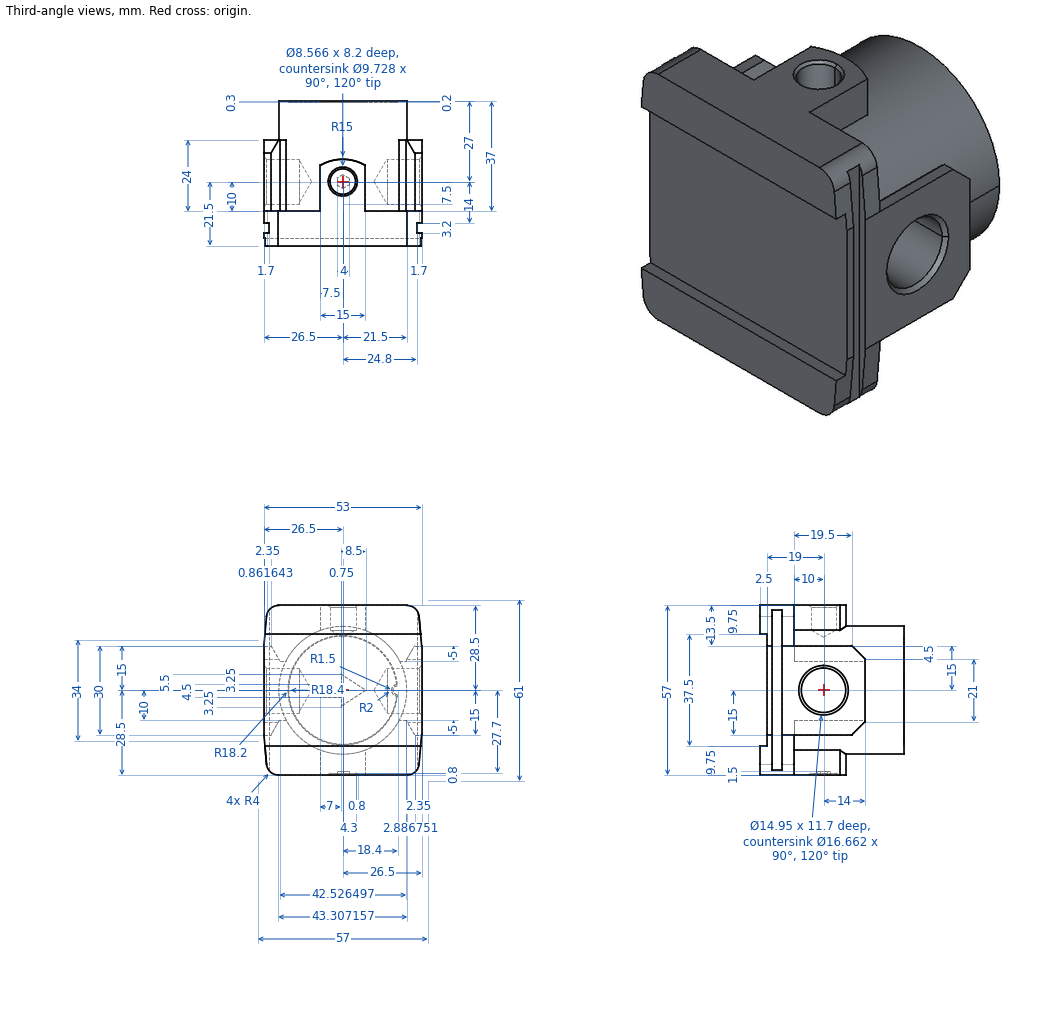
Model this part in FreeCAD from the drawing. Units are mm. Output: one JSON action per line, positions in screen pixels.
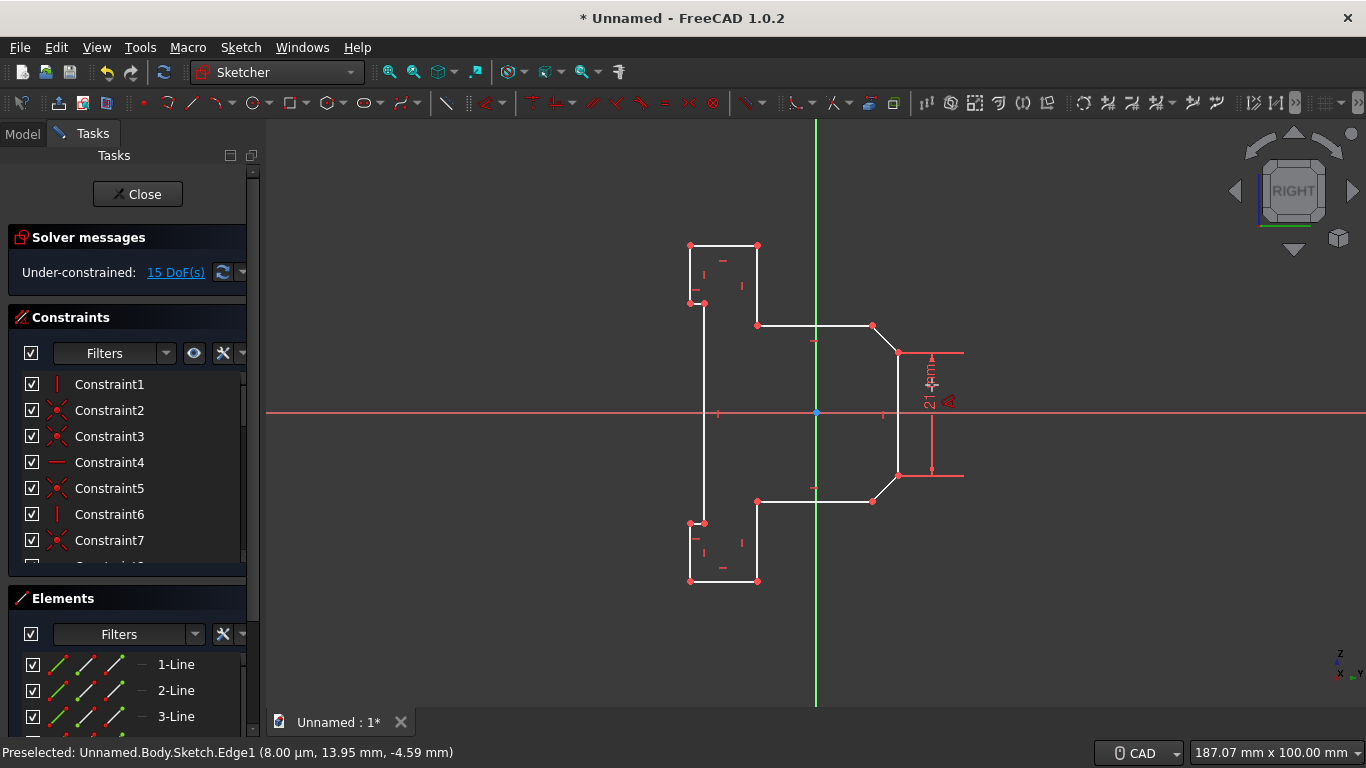
{"action": "scroll", "coordinate": [697, 304], "scroll_direction": "up", "scroll_amount": 5}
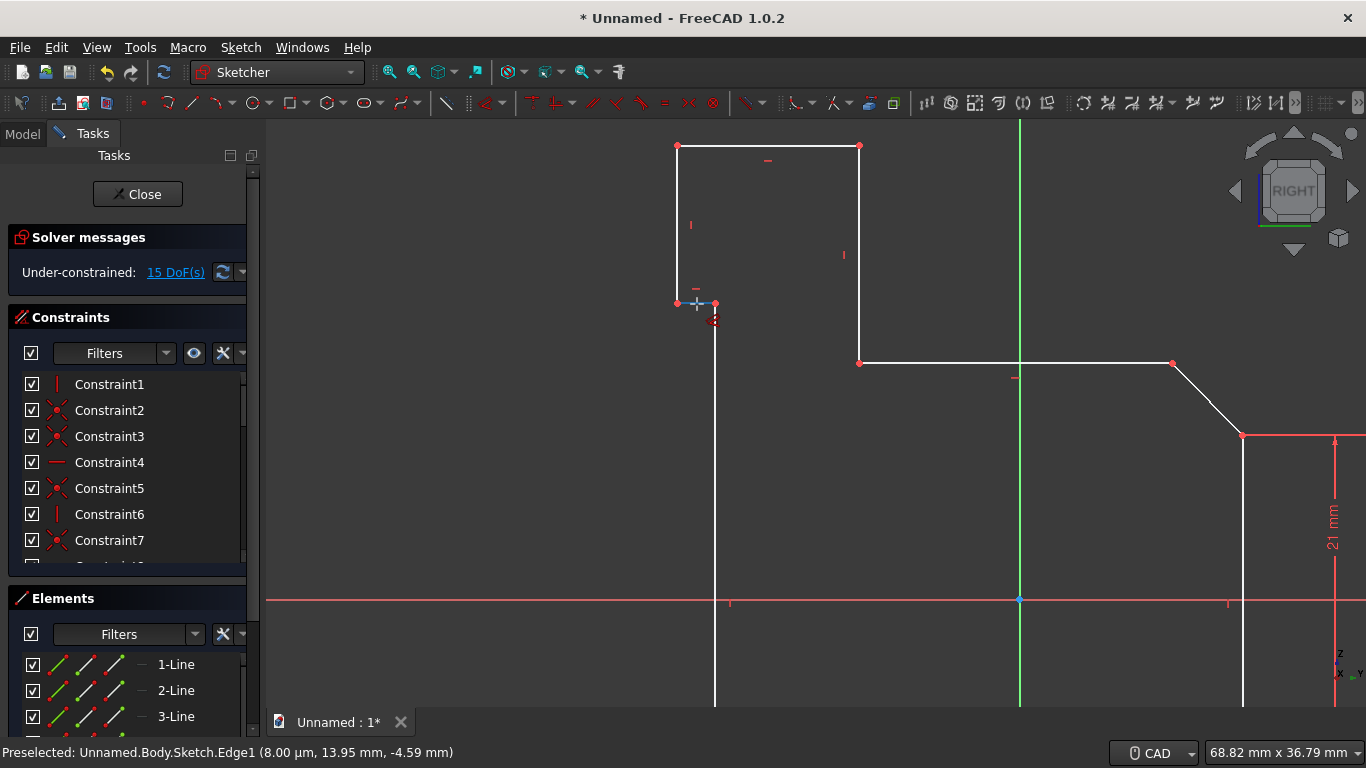
{"action": "left_click", "coordinate": [696, 303]}
{"action": "left_click", "coordinate": [696, 269]}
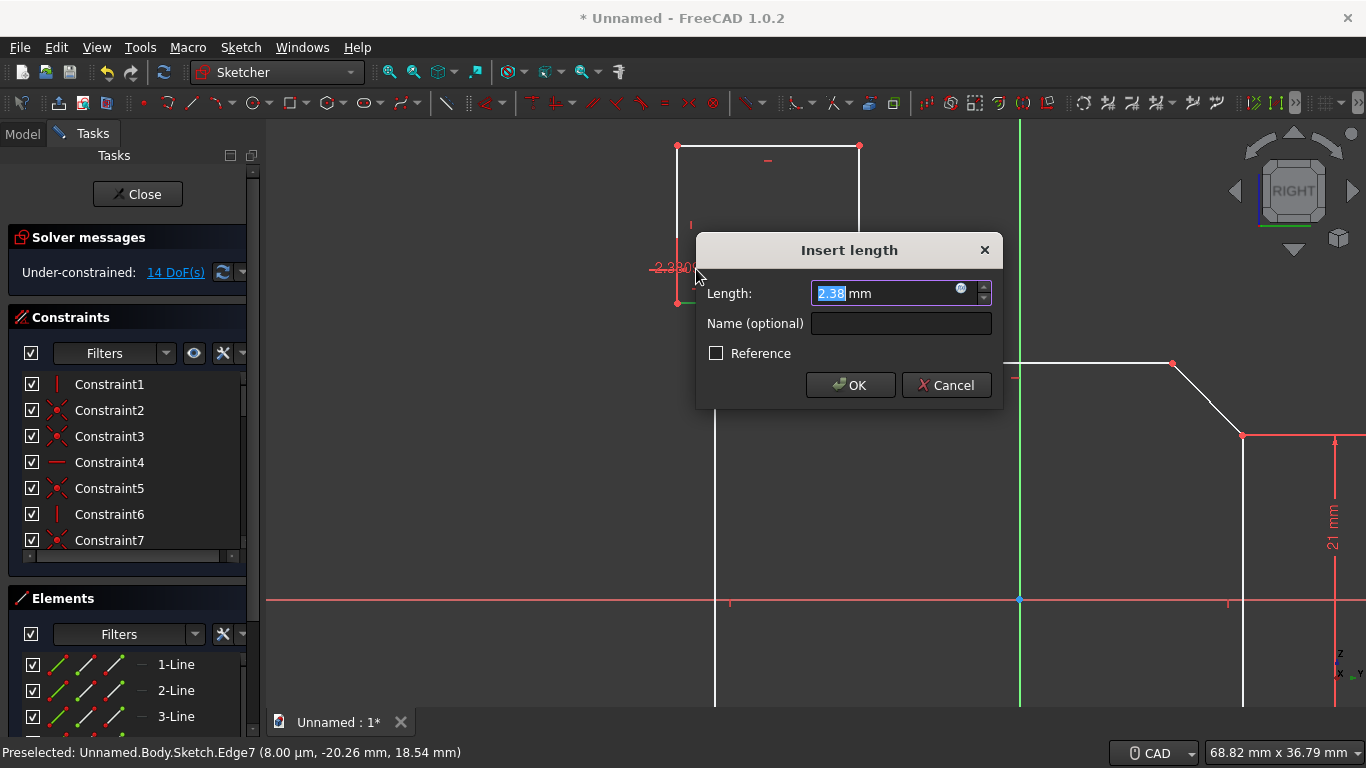
{"action": "type", "text": "2.5"}
{"action": "key", "text": "Return"}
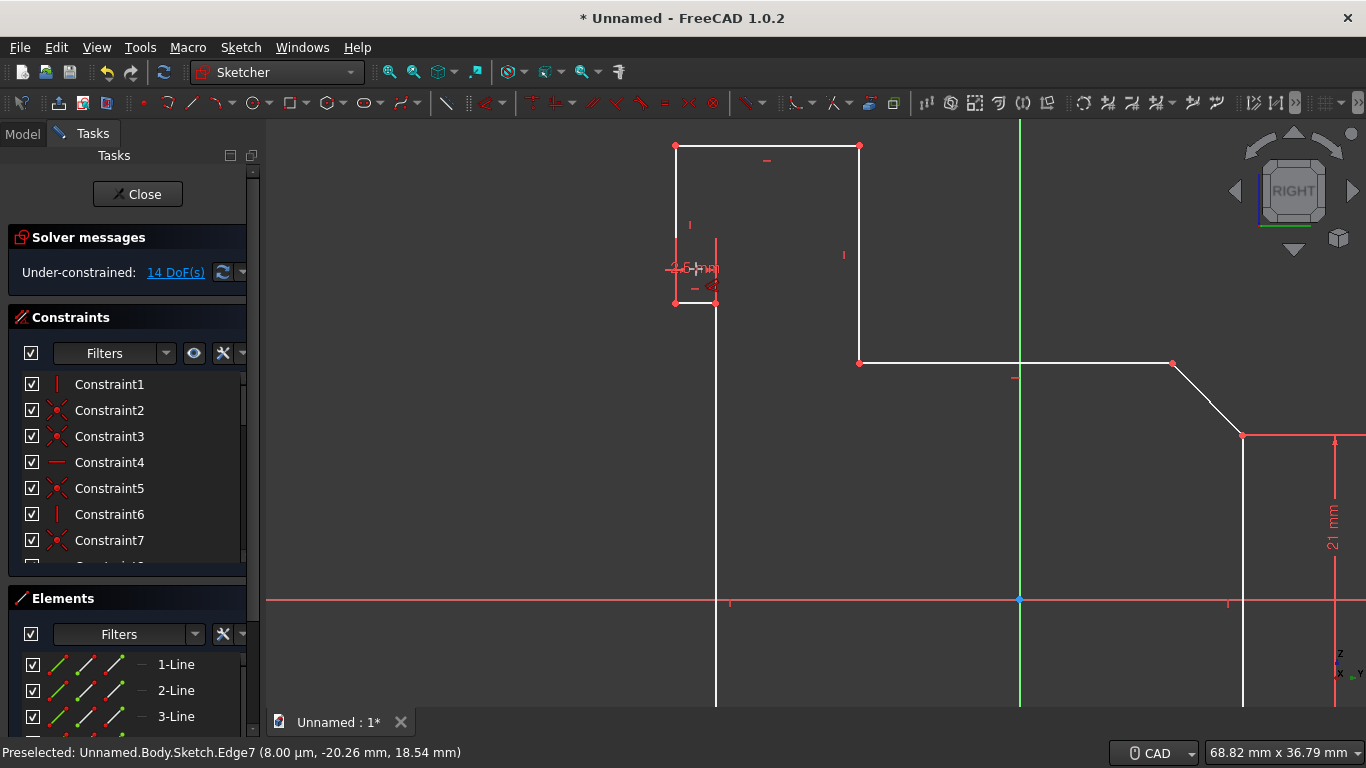
{"action": "scroll", "coordinate": [574, 261], "scroll_direction": "down", "scroll_amount": 4}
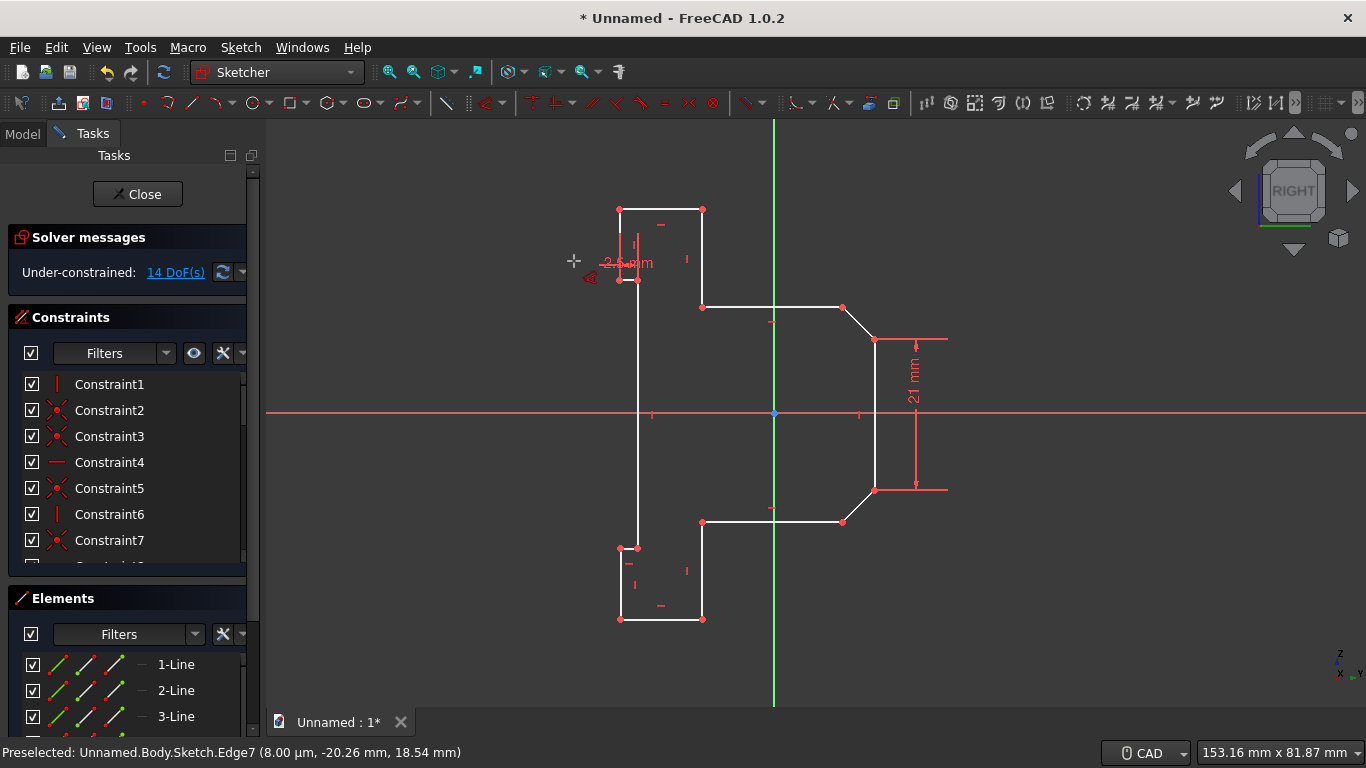
{"action": "scroll", "coordinate": [633, 549], "scroll_direction": "up", "scroll_amount": 5}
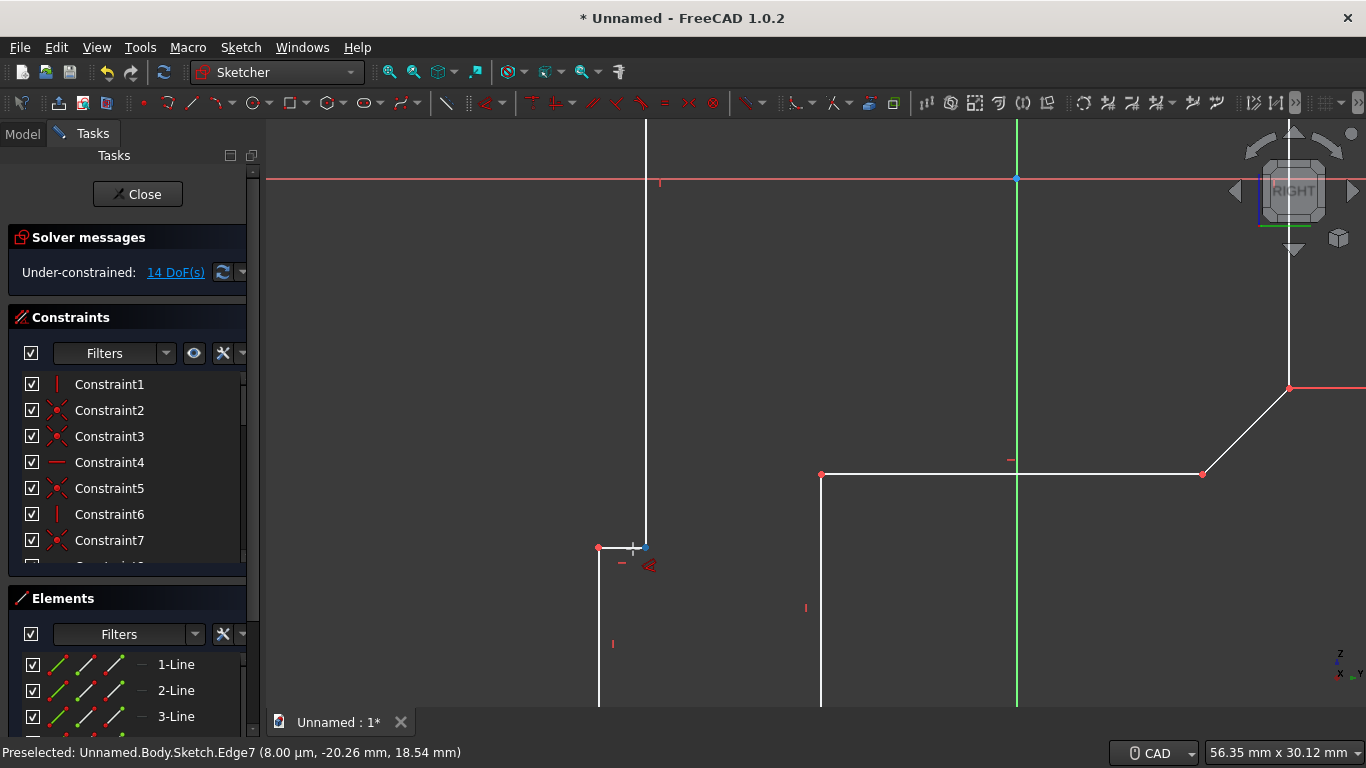
{"action": "left_click", "coordinate": [631, 548]}
{"action": "left_click", "coordinate": [622, 582]}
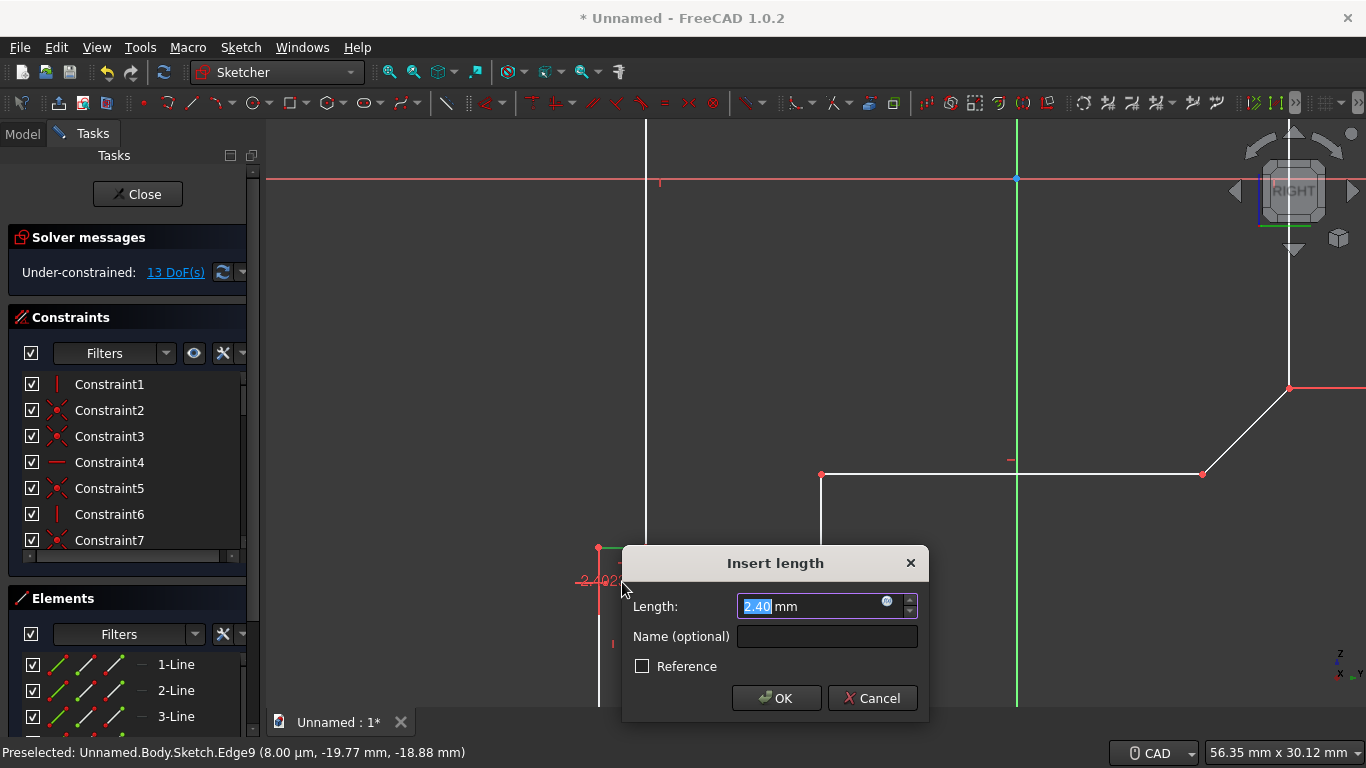
{"action": "type", "text": "2.5"}
{"action": "key", "text": "Return"}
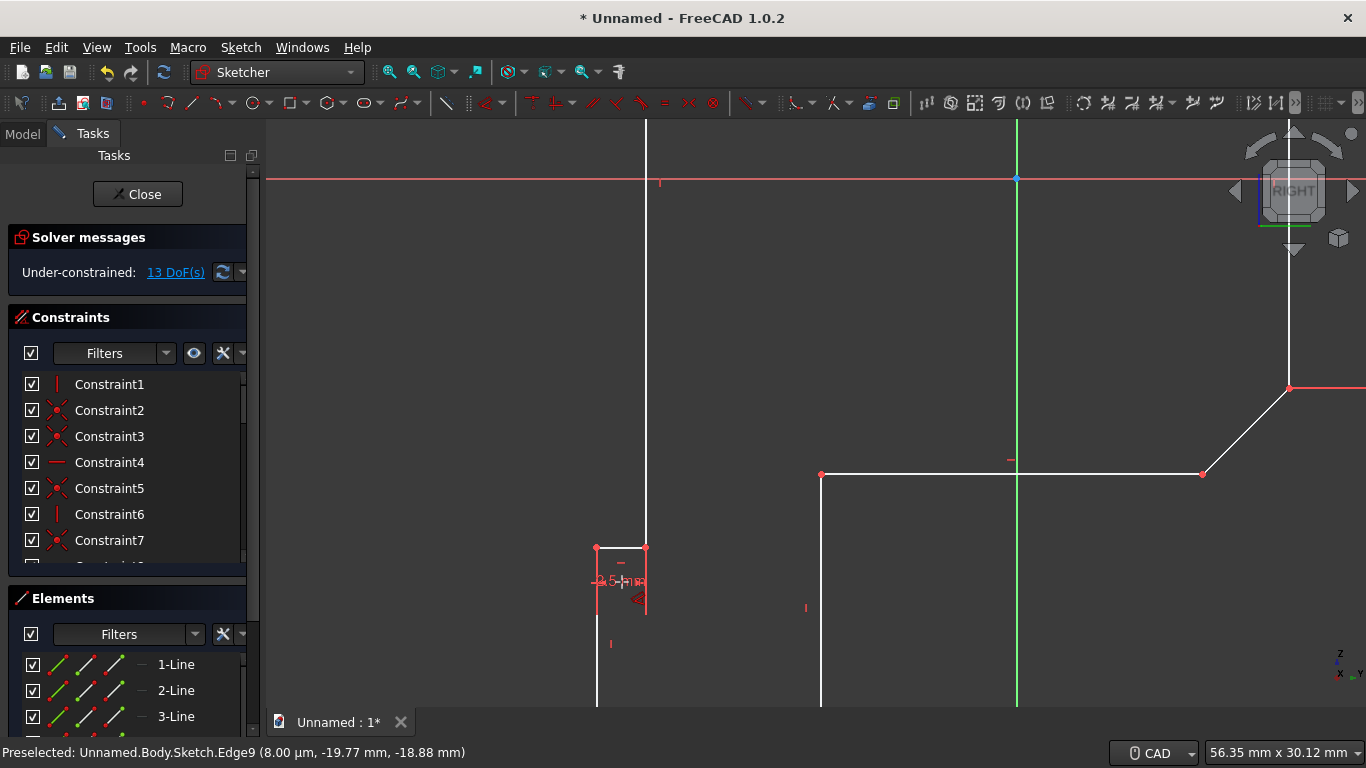
{"action": "scroll", "coordinate": [633, 549], "scroll_direction": "down", "scroll_amount": 5}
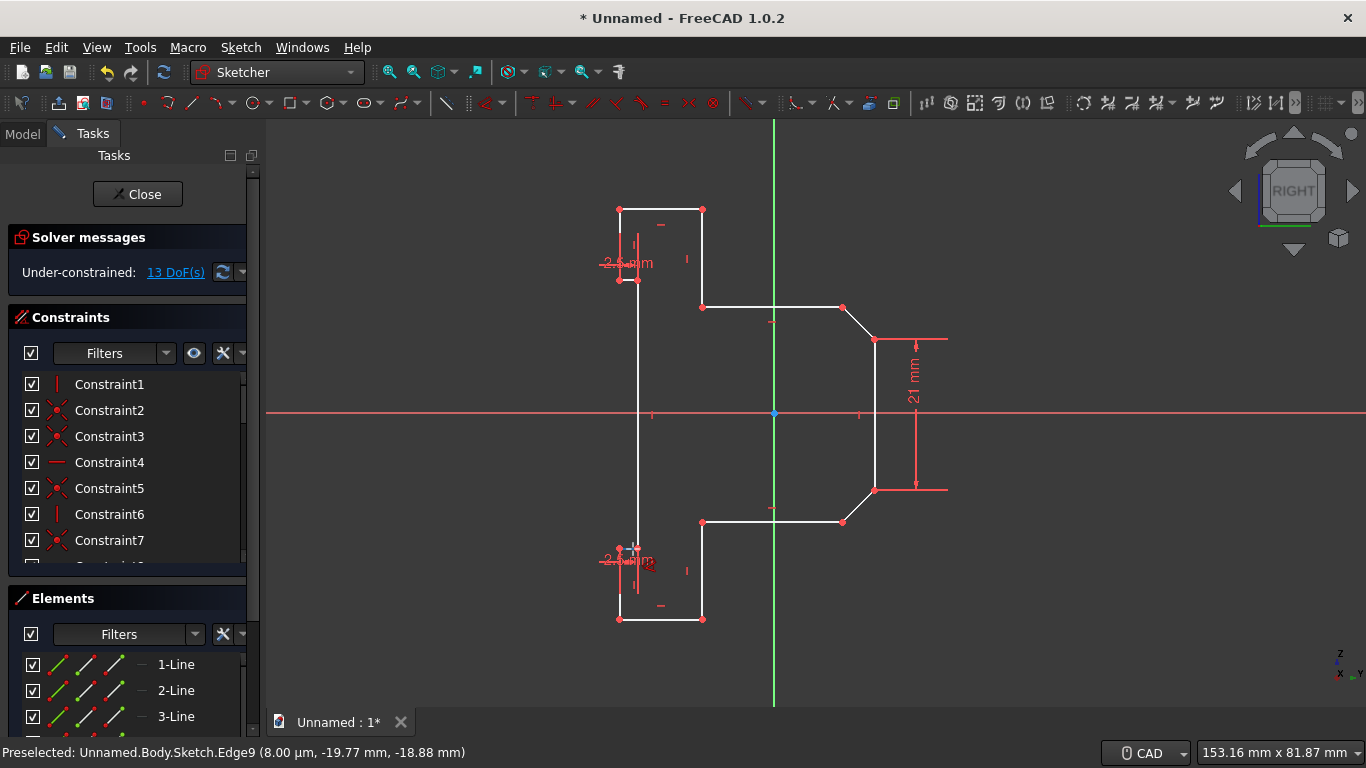
{"action": "left_click", "coordinate": [875, 490]}
{"action": "left_click", "coordinate": [860, 524]}